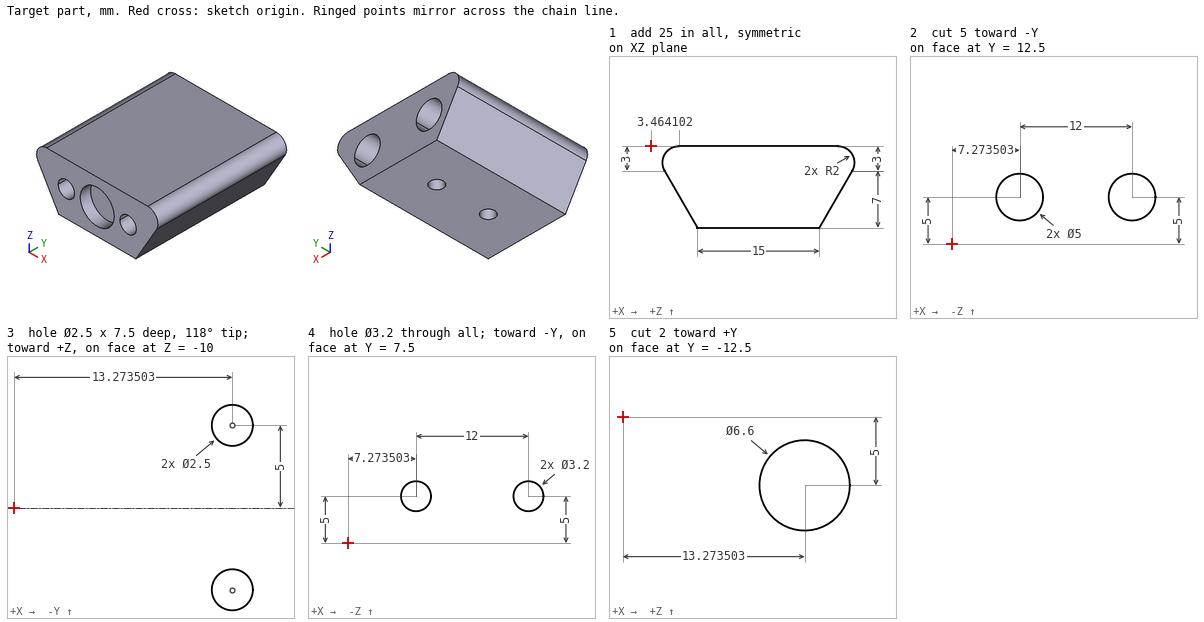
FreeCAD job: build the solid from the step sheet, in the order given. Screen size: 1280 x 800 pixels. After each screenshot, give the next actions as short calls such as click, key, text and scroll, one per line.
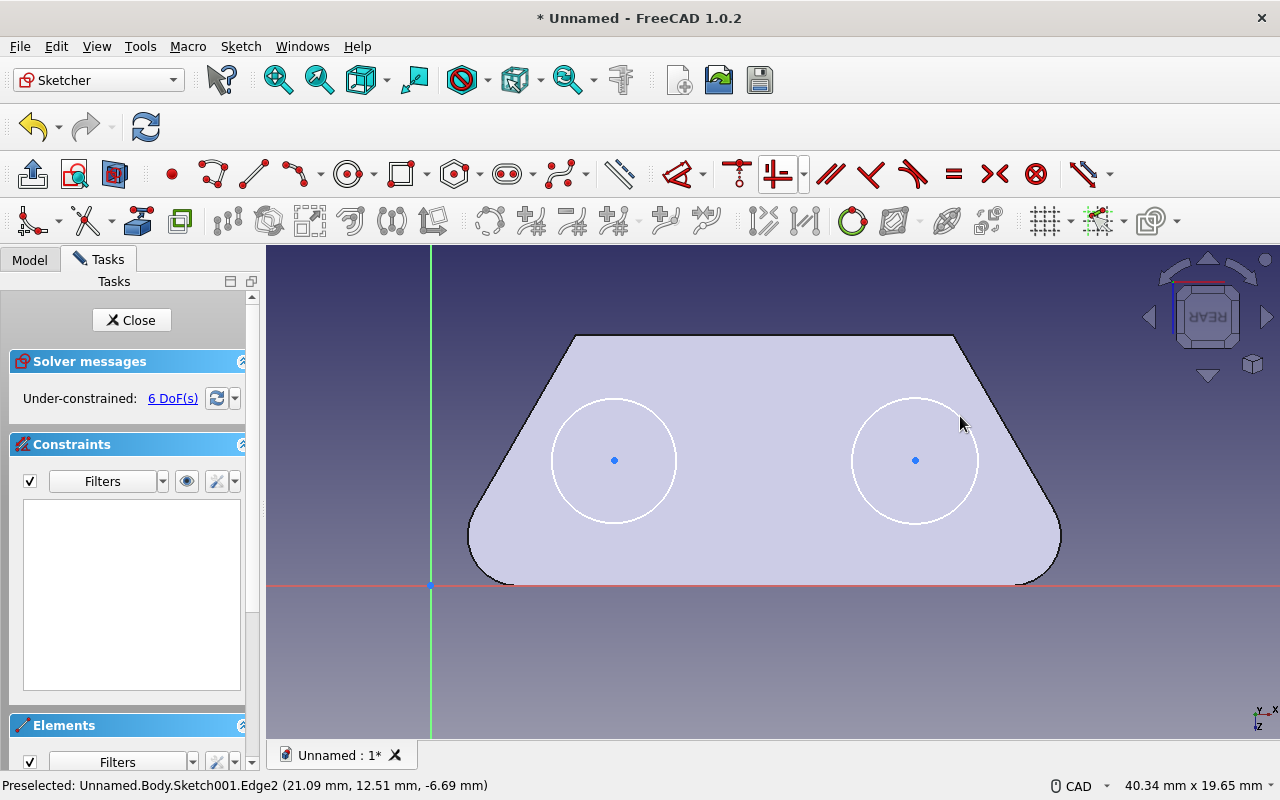
click(658, 417)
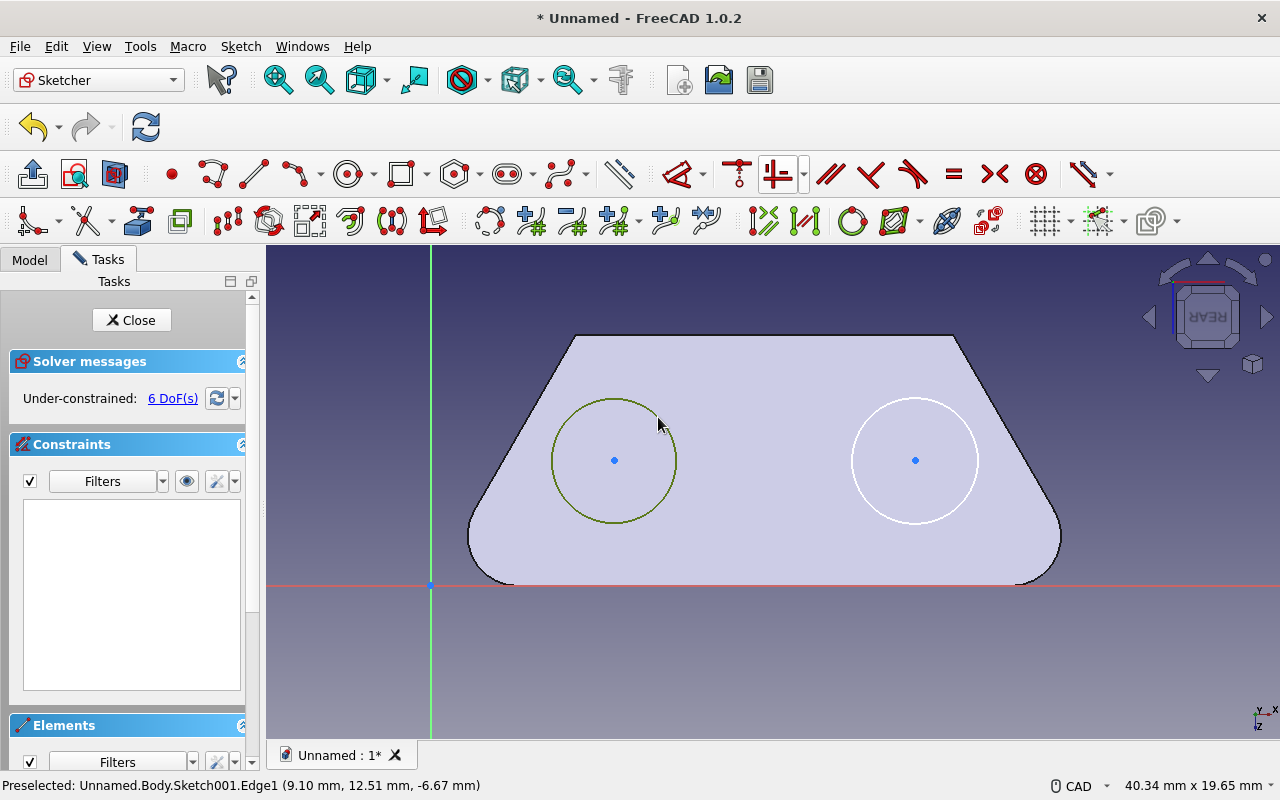
click(959, 416)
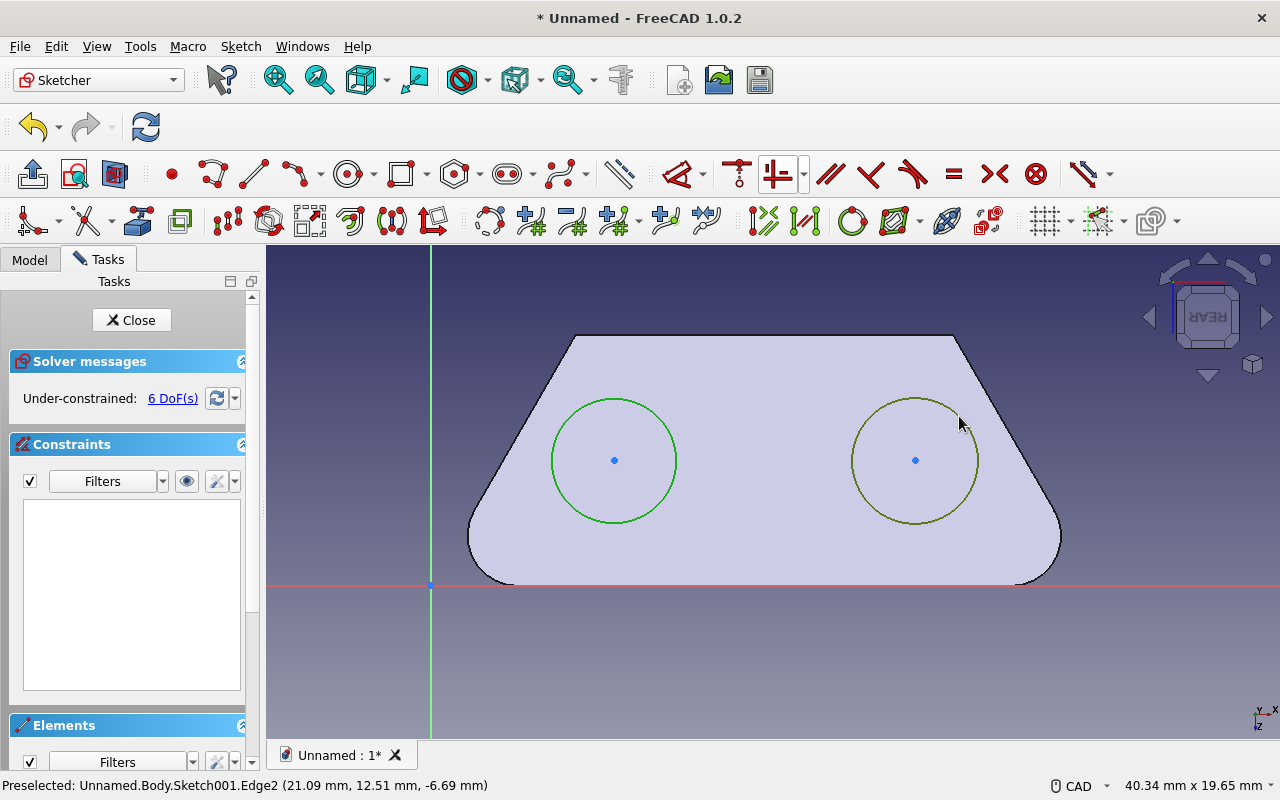
click(954, 174)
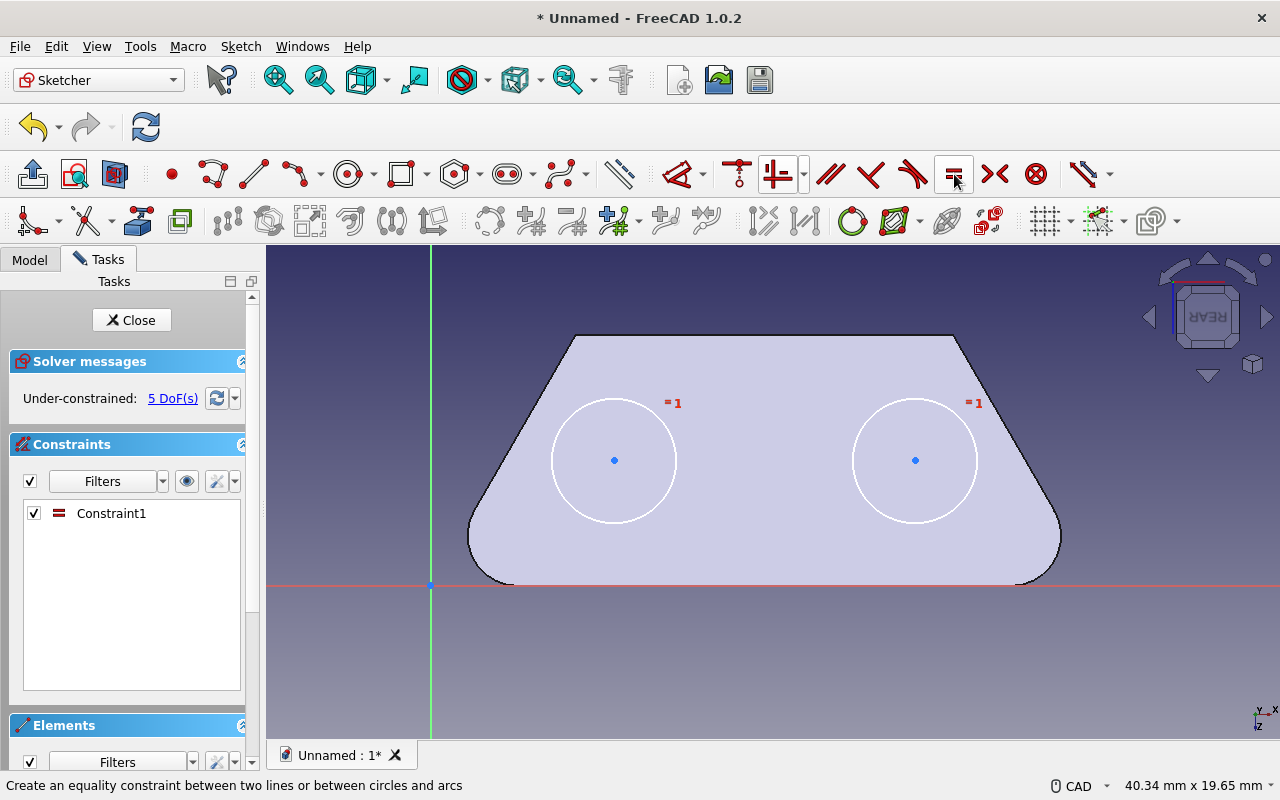
click(676, 174)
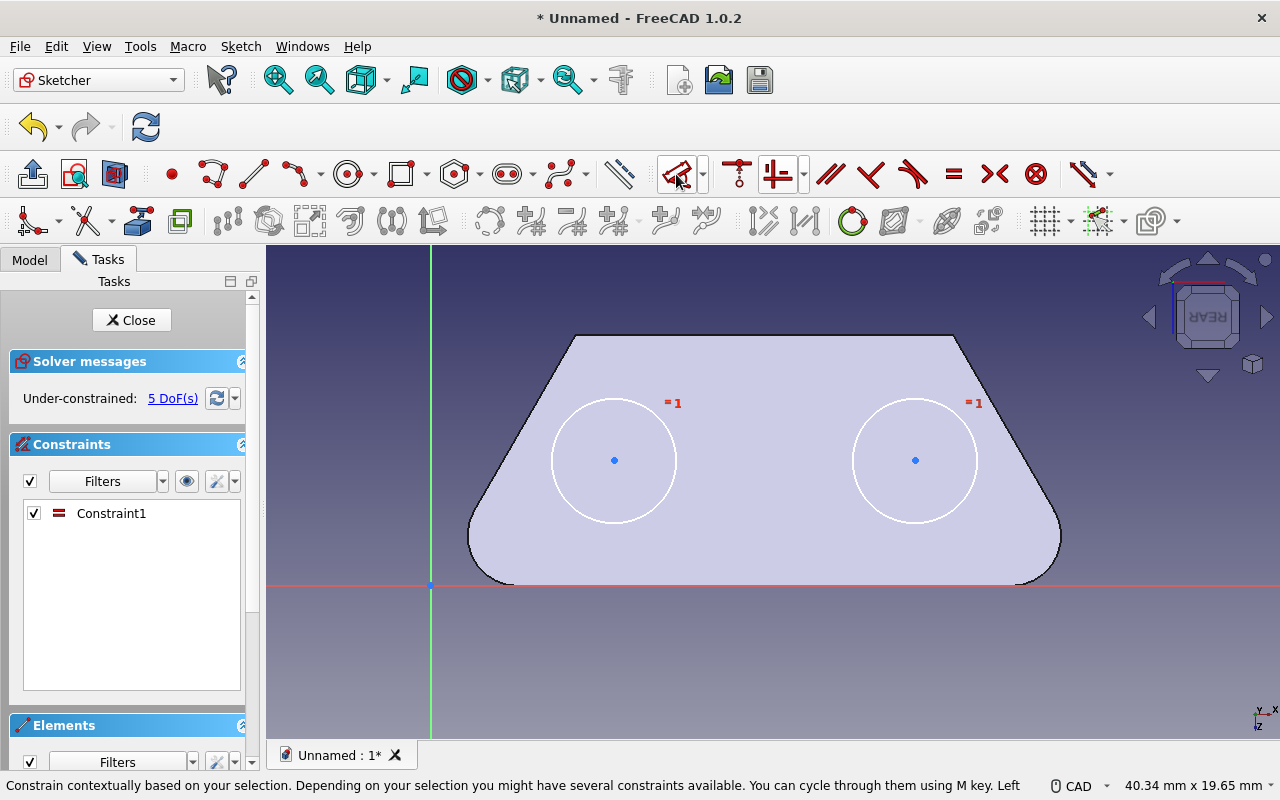
click(658, 417)
click(681, 394)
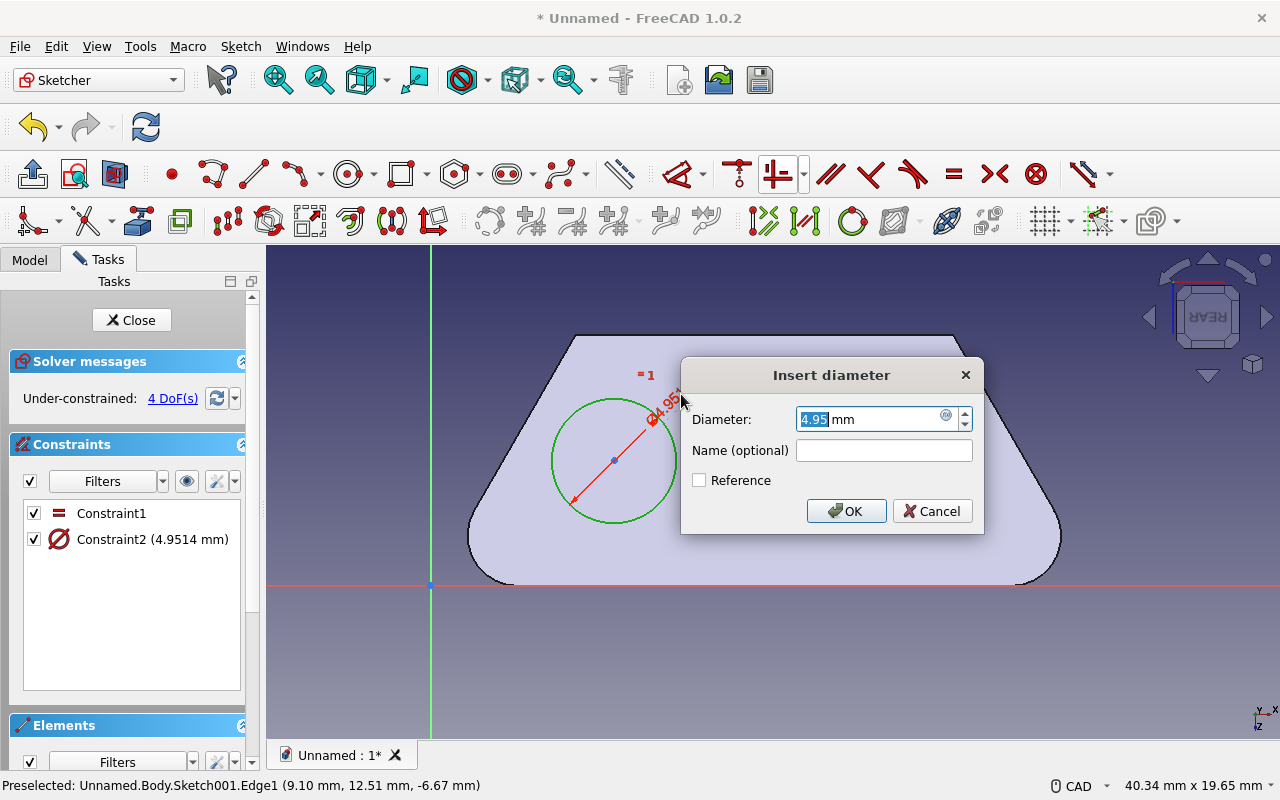
text(5)
key(Return)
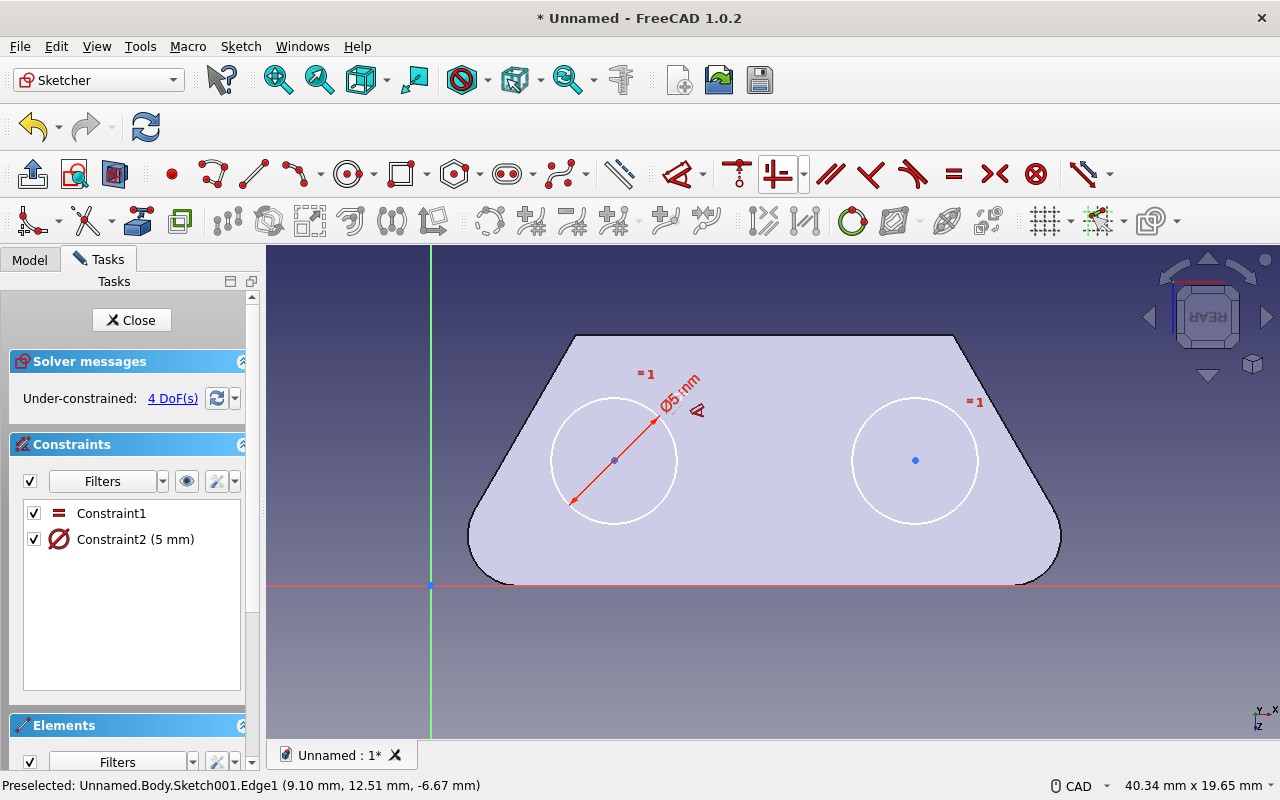
click(614, 461)
click(397, 523)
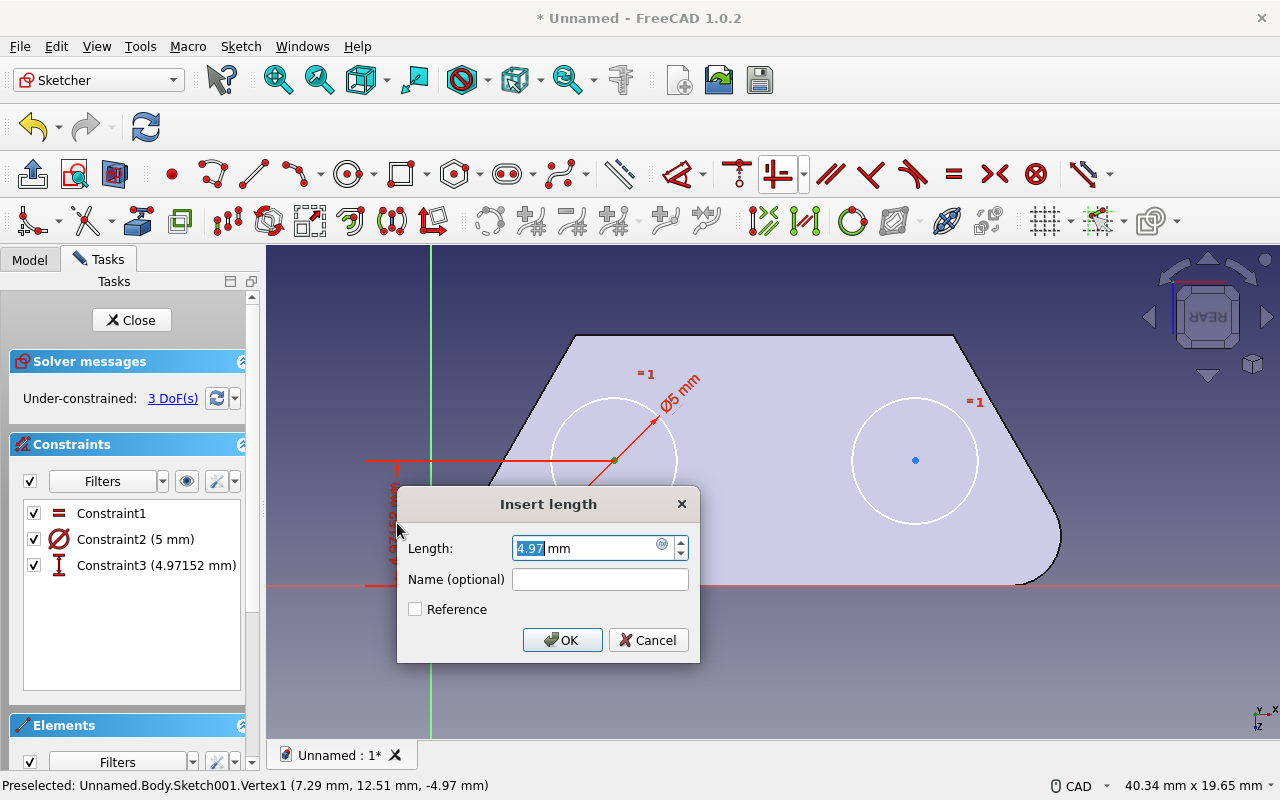
text(5)
key(Return)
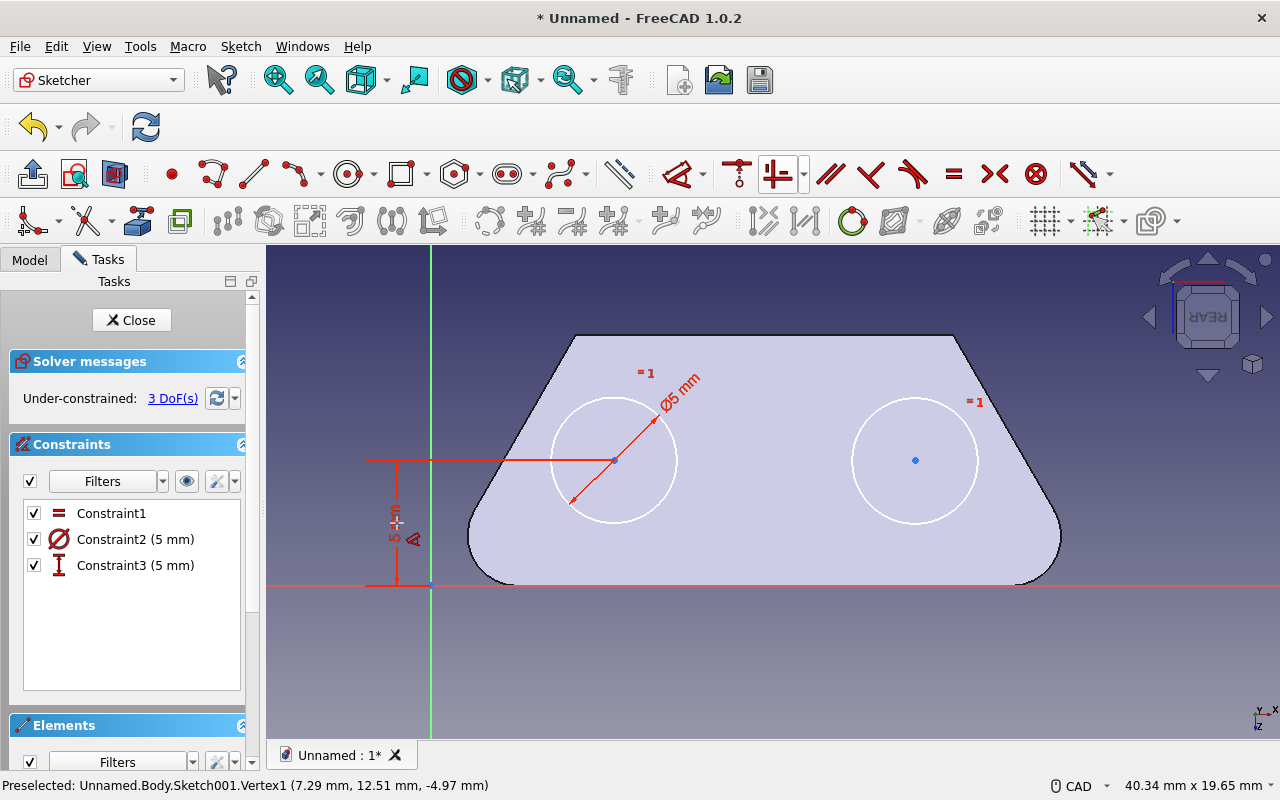
click(915, 461)
click(397, 495)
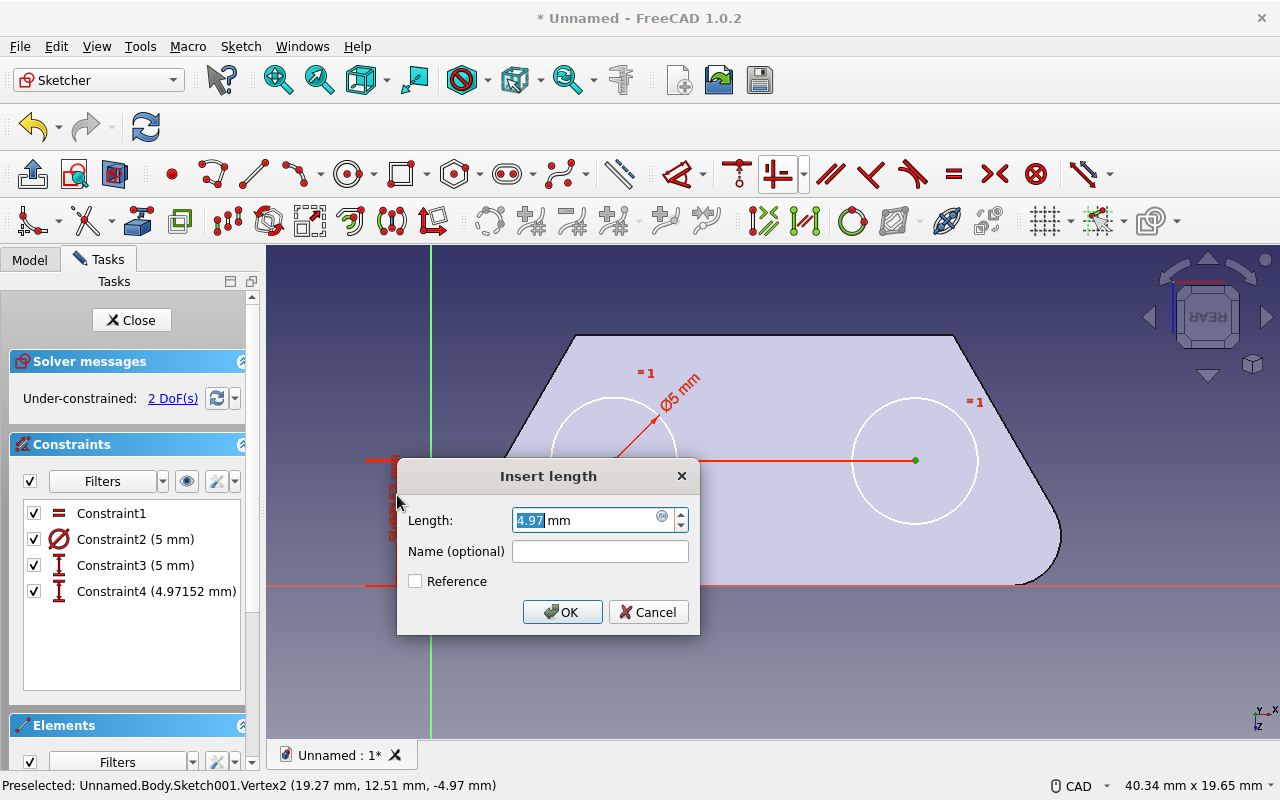
text(5)
key(Return)